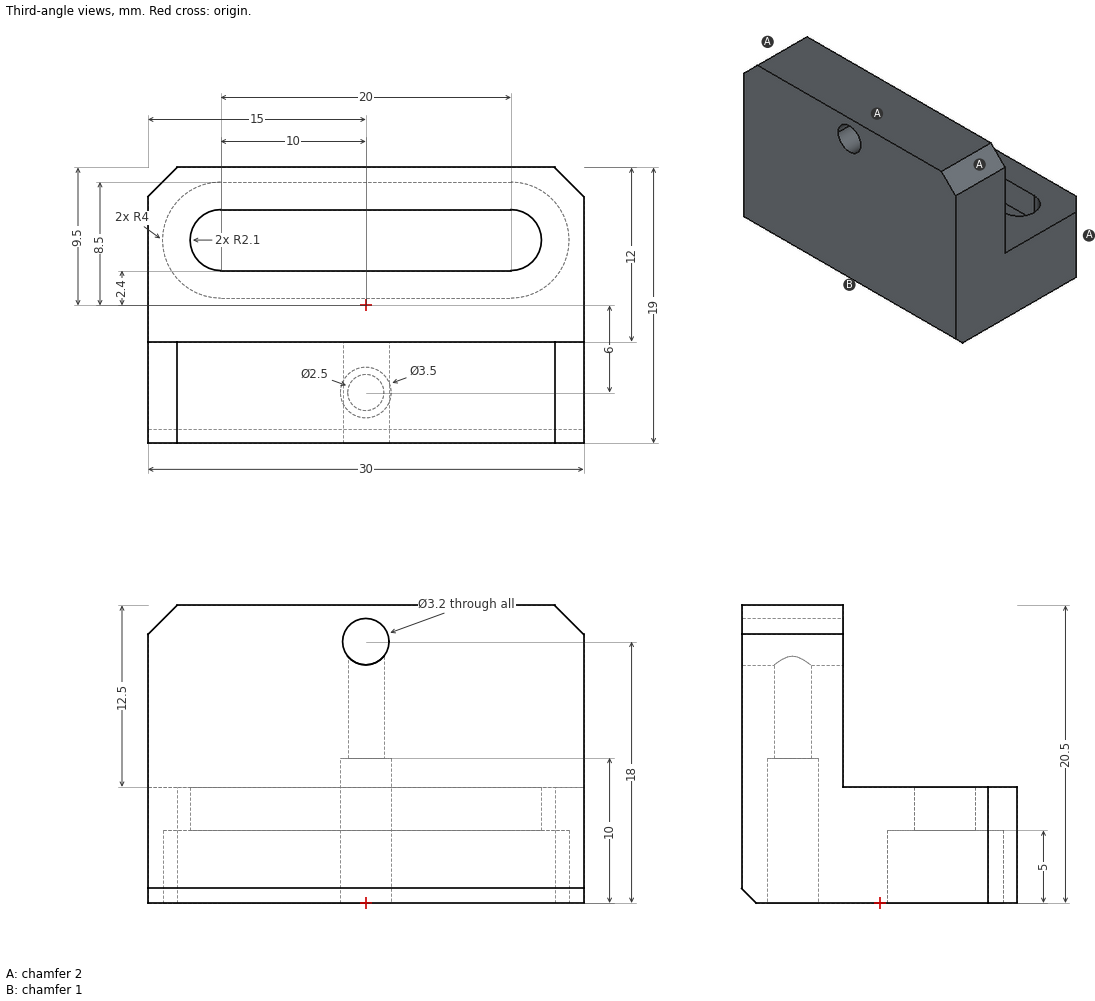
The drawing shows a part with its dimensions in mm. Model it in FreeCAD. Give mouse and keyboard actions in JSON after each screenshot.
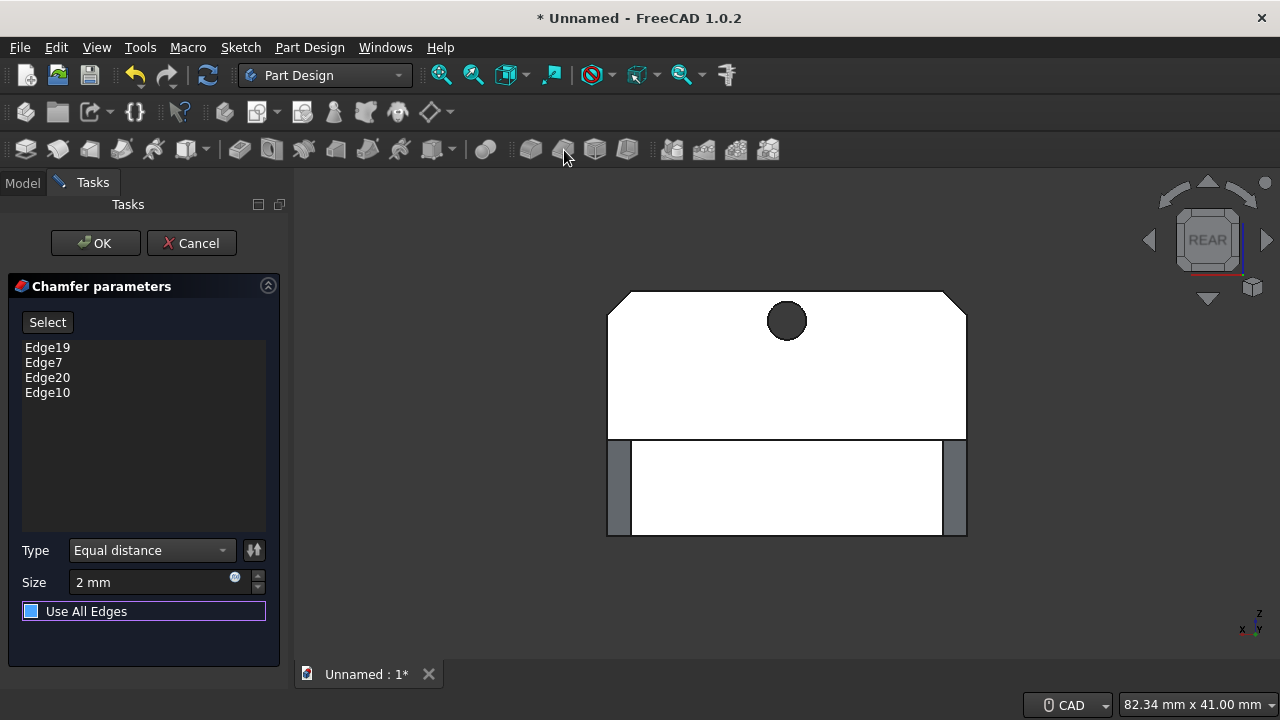
{"action": "left_click", "coordinate": [96, 243]}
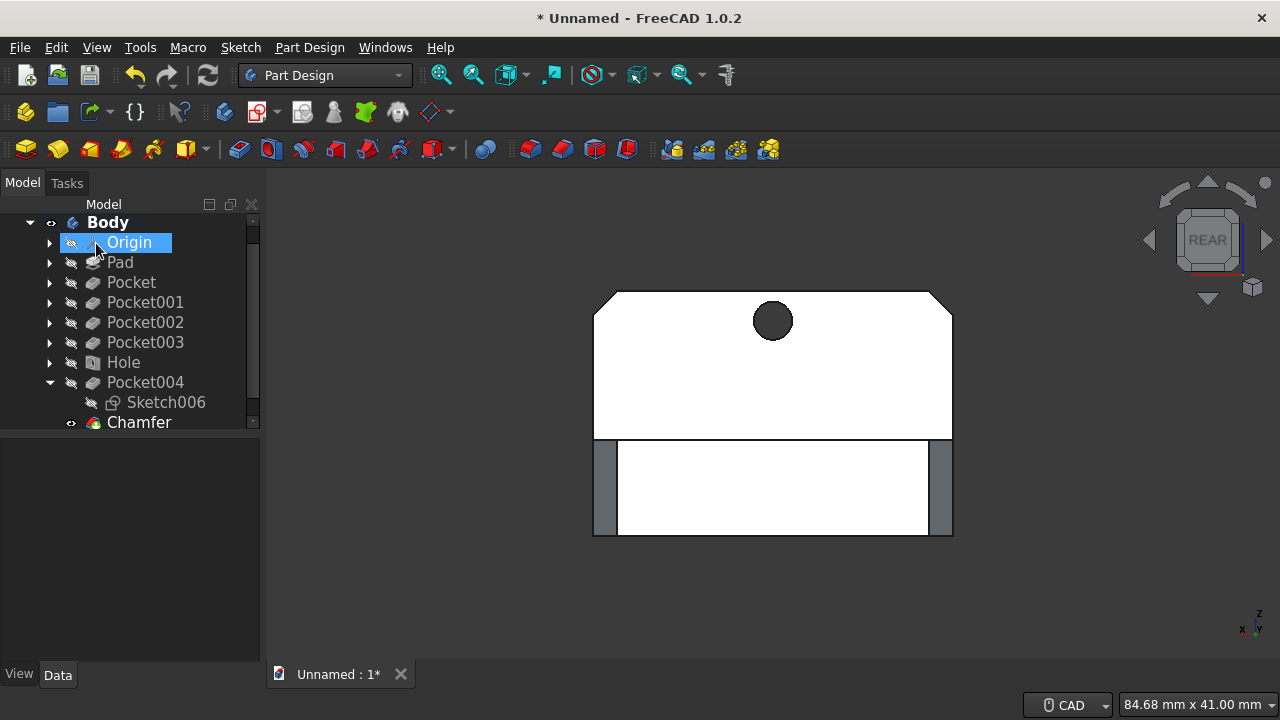
{"action": "key", "text": "0"}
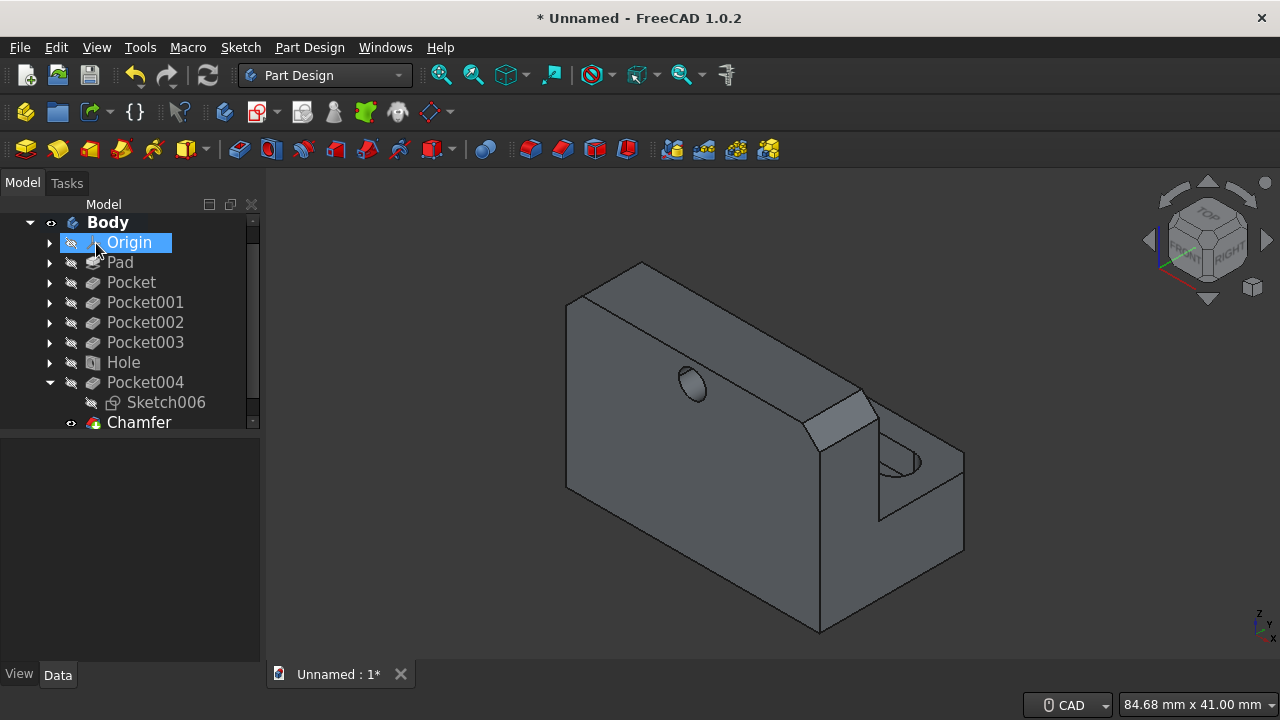
{"action": "key", "text": "2"}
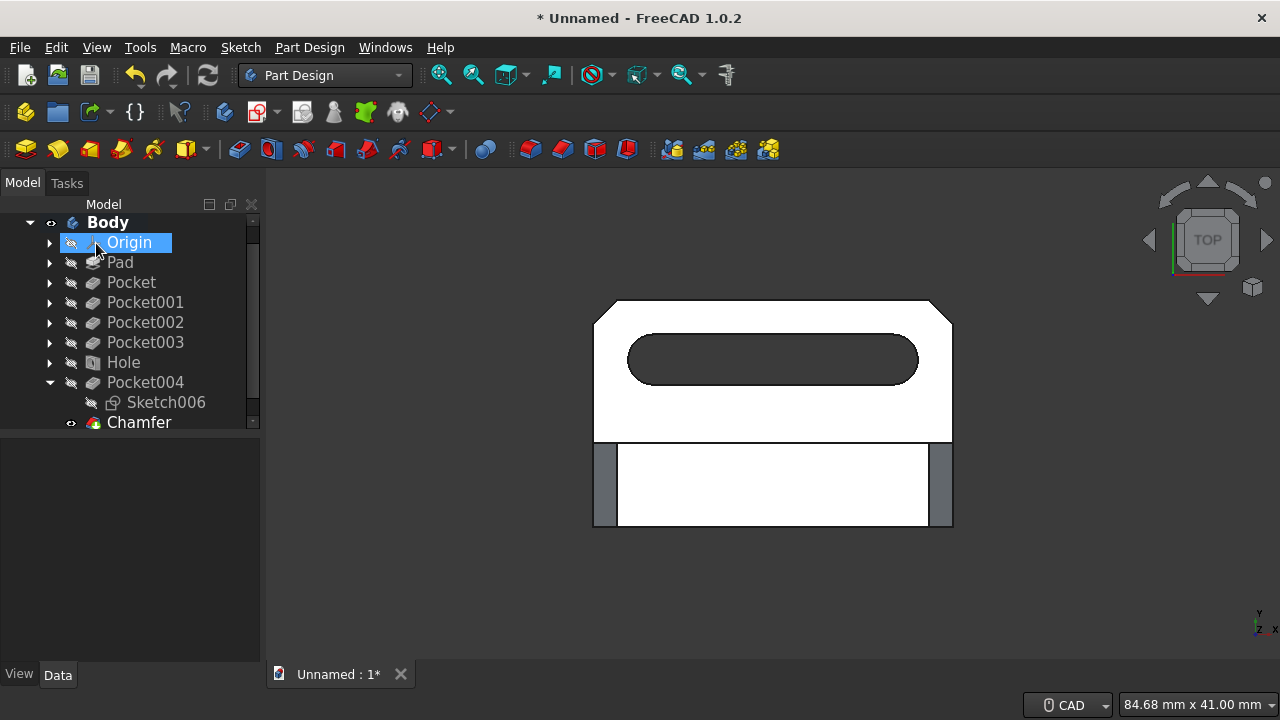
{"action": "key", "text": "1"}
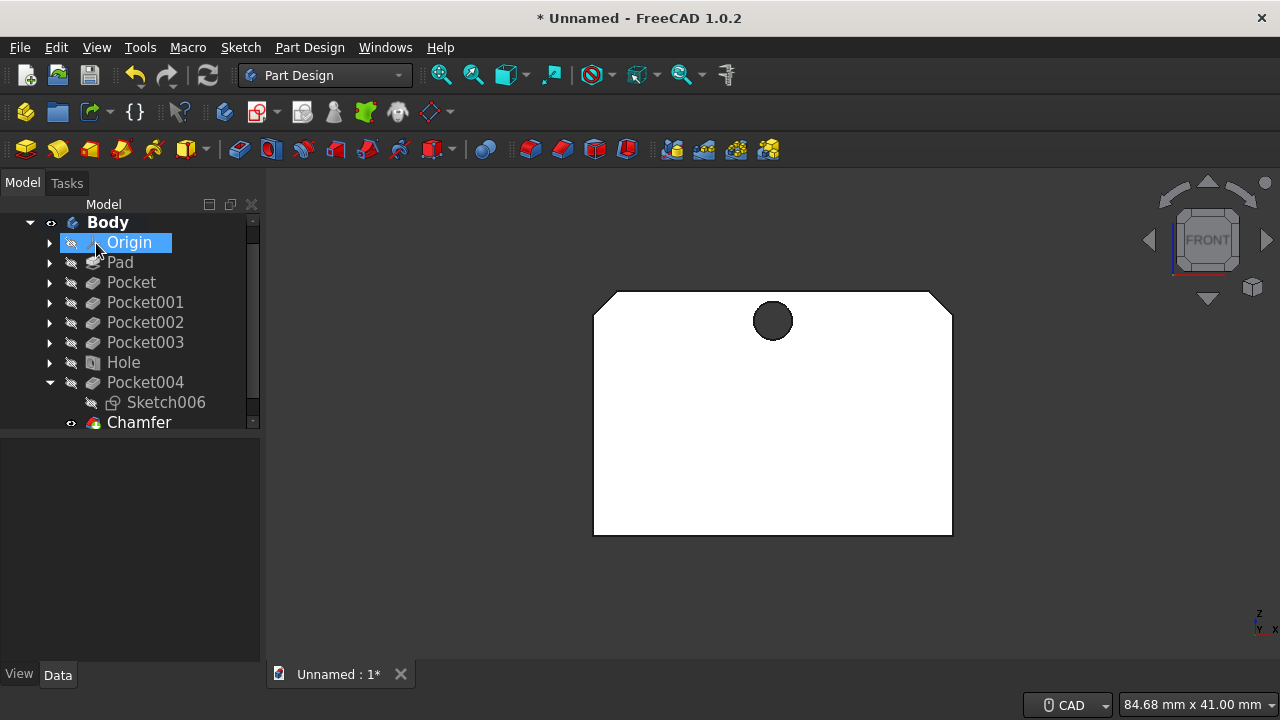
{"action": "left_click", "coordinate": [773, 535]}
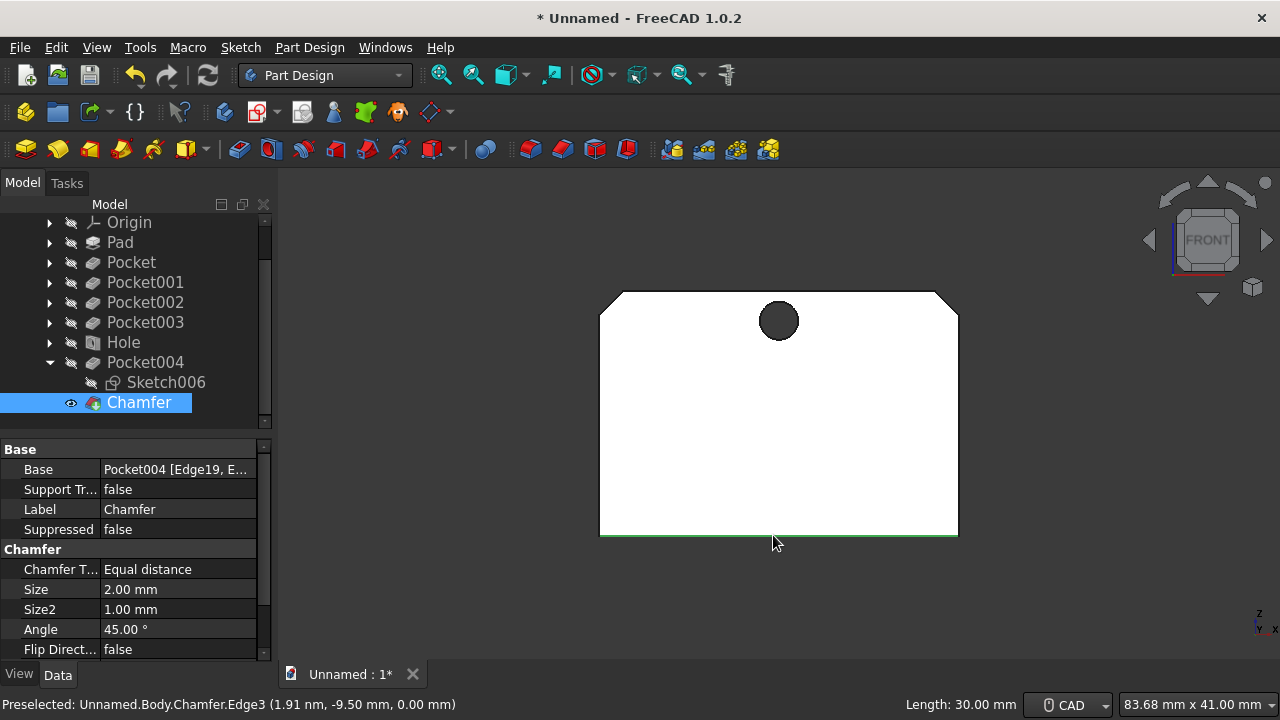
{"action": "left_click", "coordinate": [564, 150]}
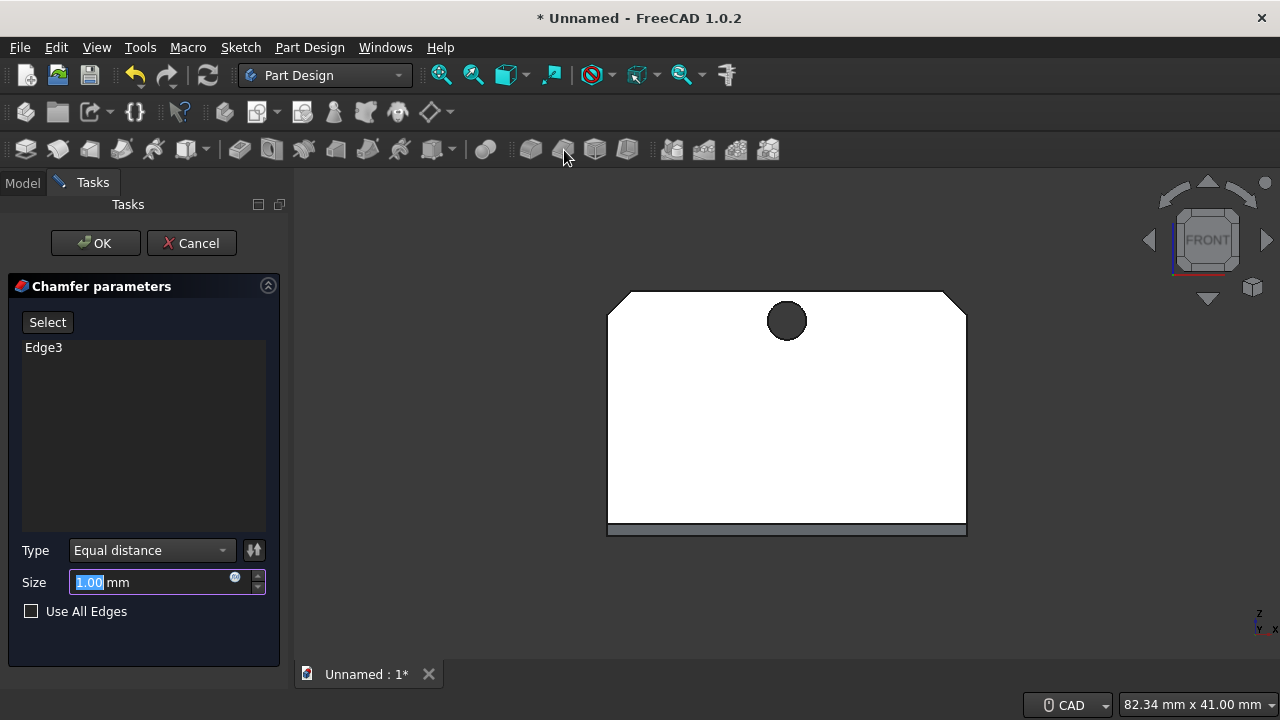
{"action": "type", "text": "1"}
{"action": "key", "text": "Tab"}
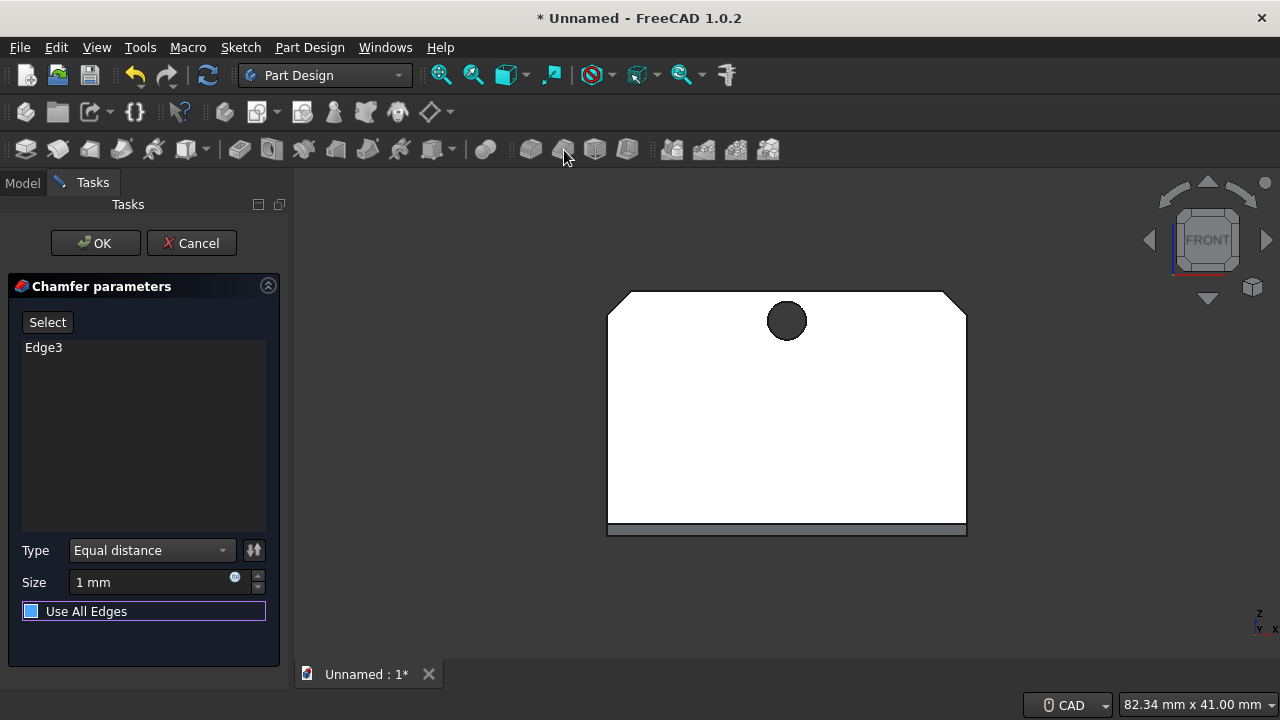
{"action": "left_click", "coordinate": [96, 243]}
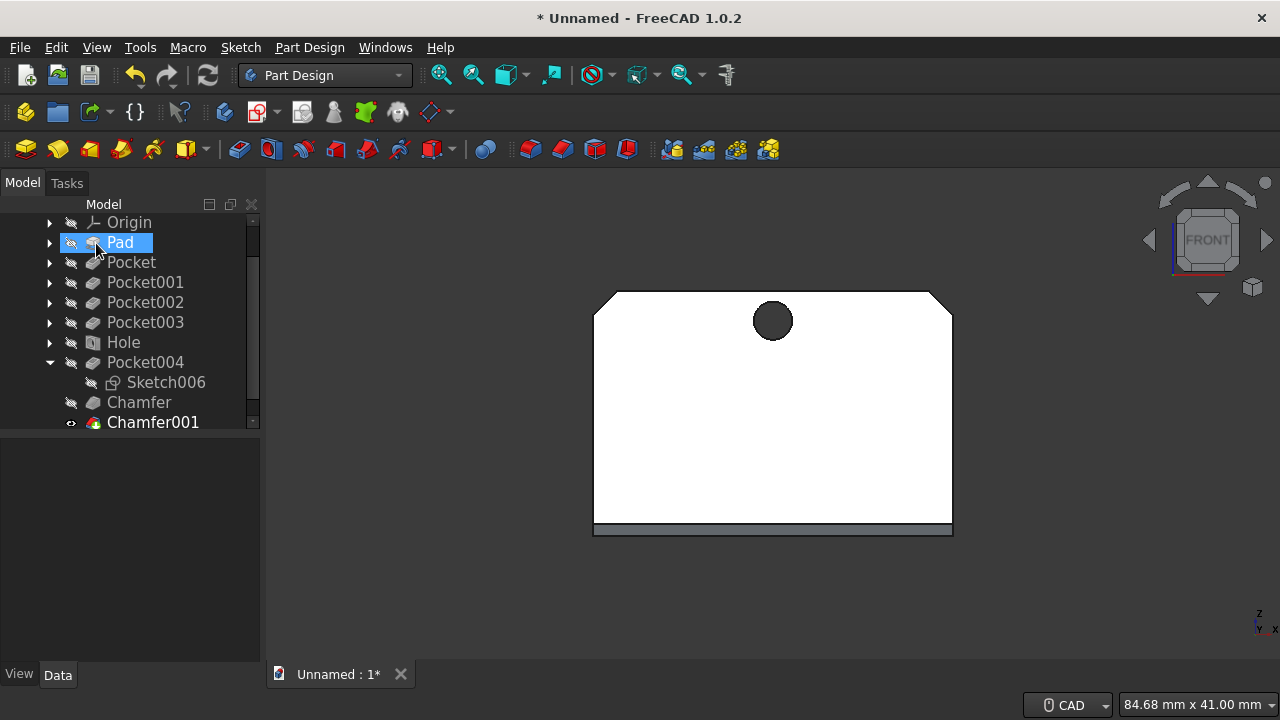
{"action": "key", "text": "0"}